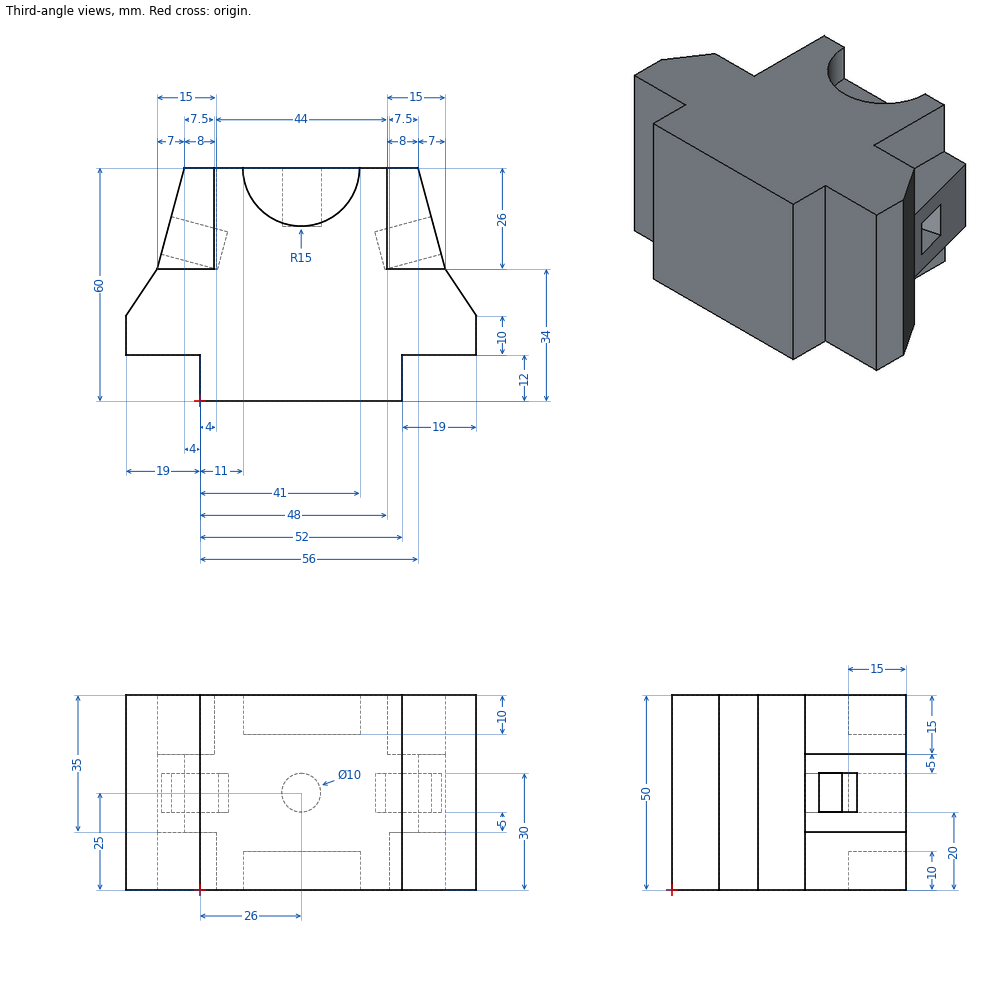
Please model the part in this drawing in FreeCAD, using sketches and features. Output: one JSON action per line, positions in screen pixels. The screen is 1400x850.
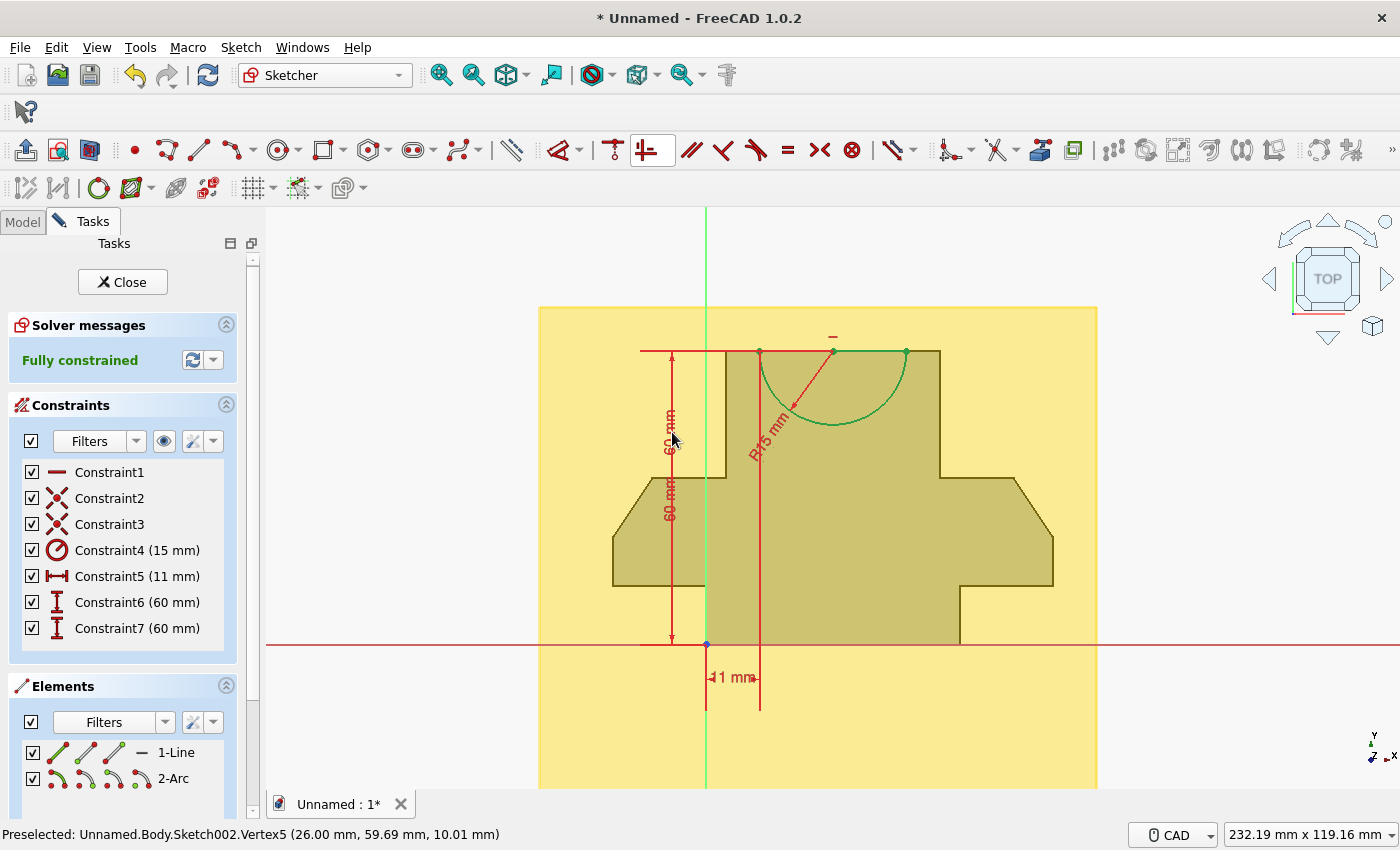
{"action": "left_click", "coordinate": [123, 282]}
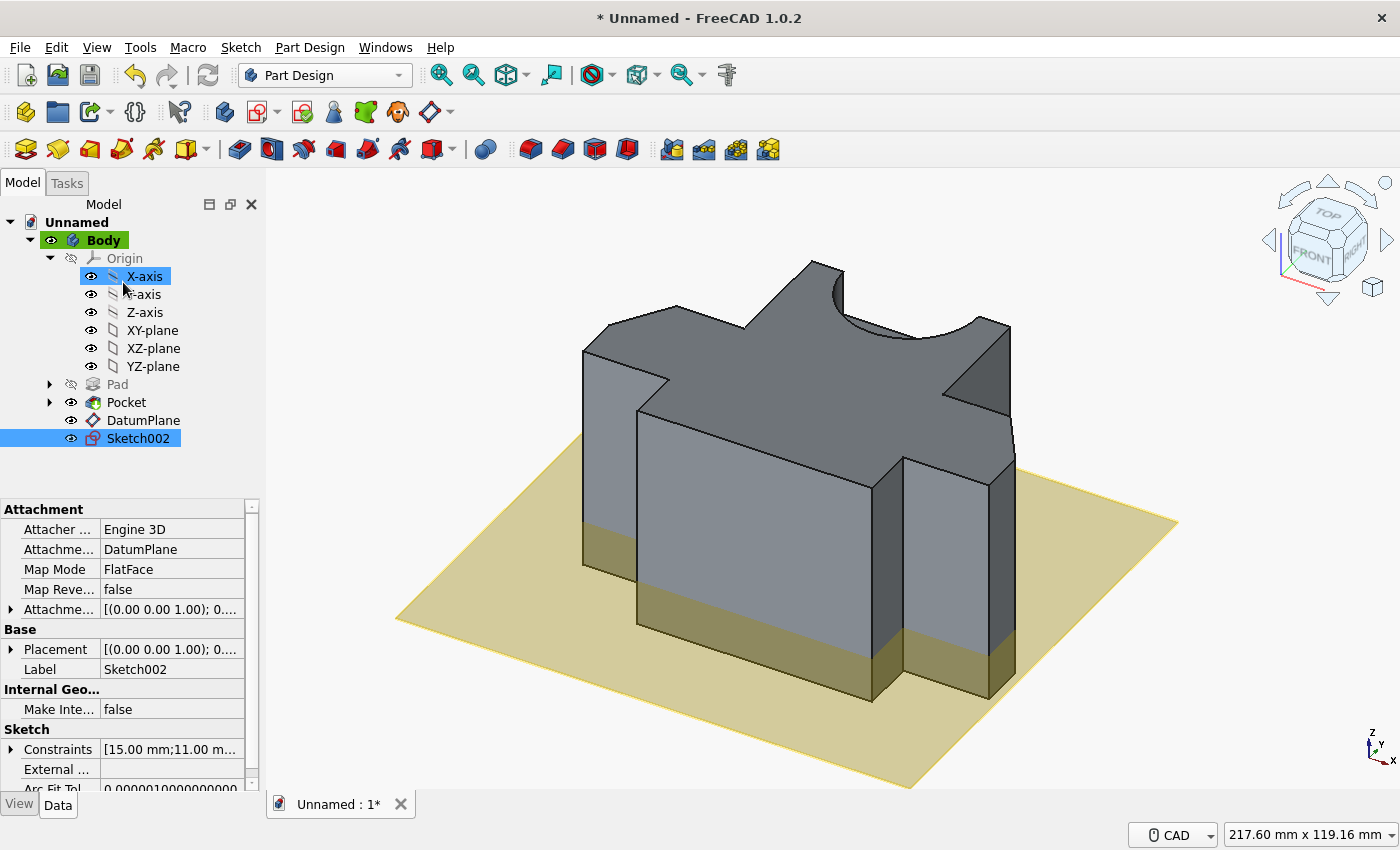
{"action": "left_click", "coordinate": [240, 150]}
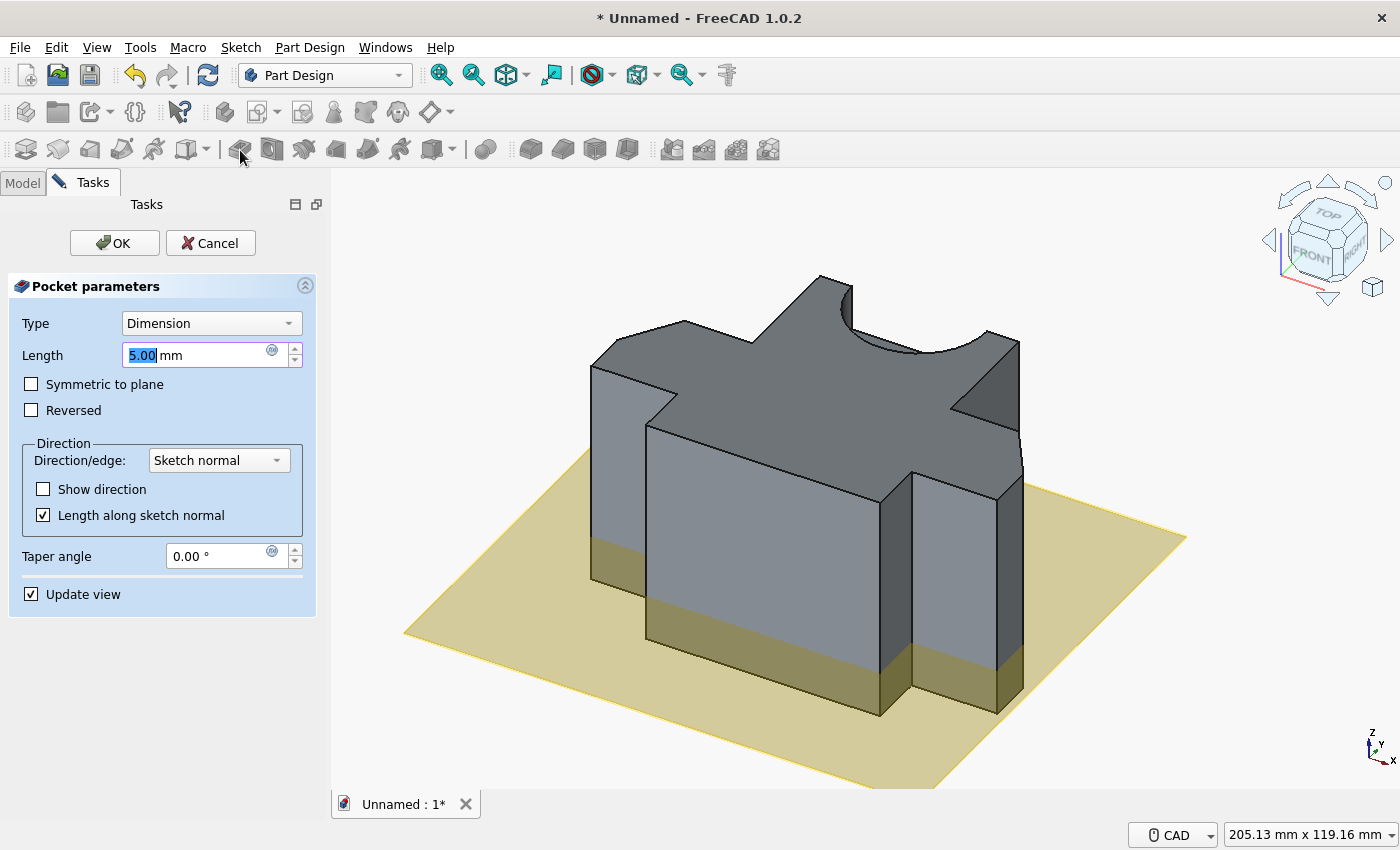
{"action": "type", "text": "10"}
{"action": "key", "text": "Tab"}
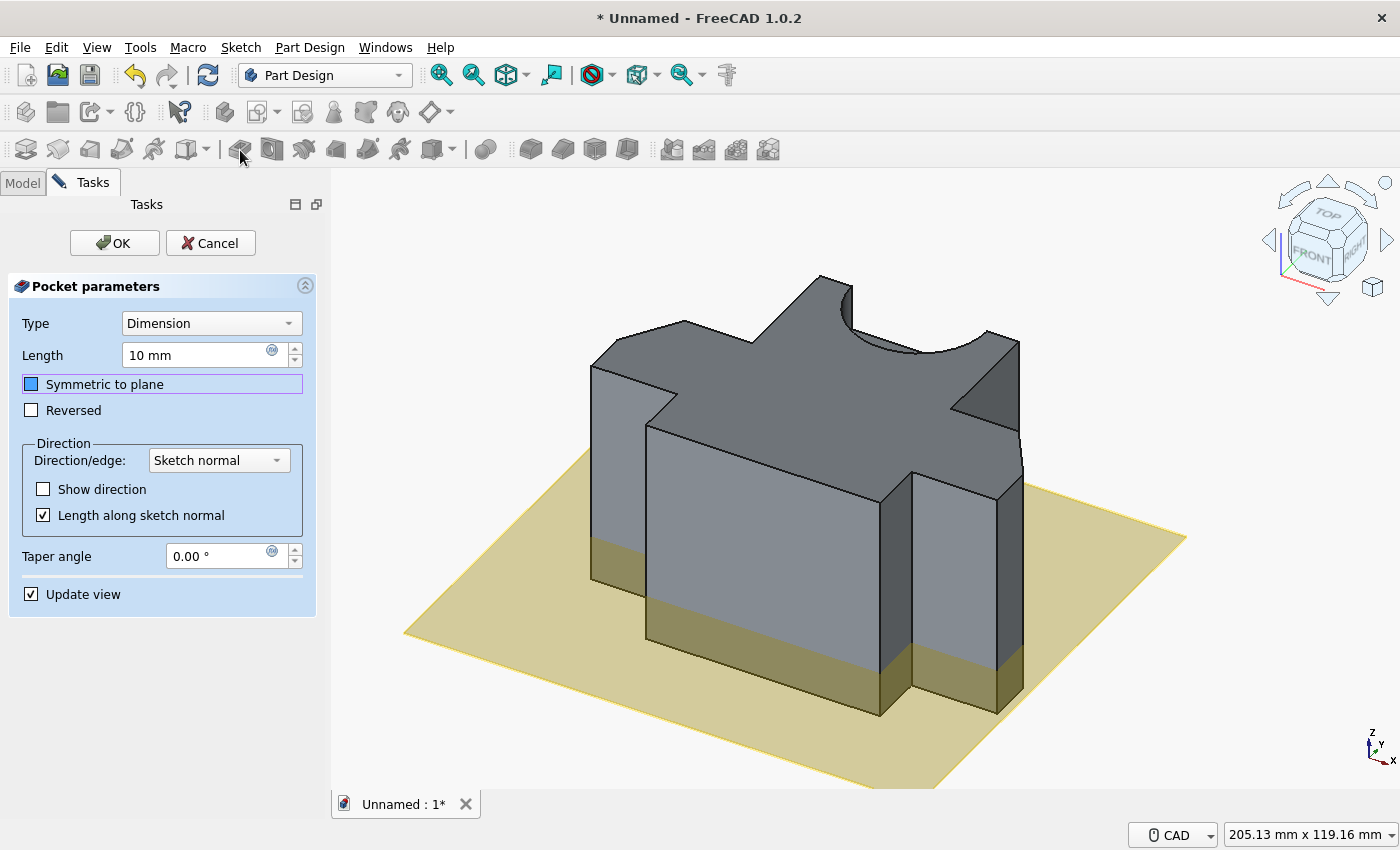
{"action": "left_click", "coordinate": [115, 243]}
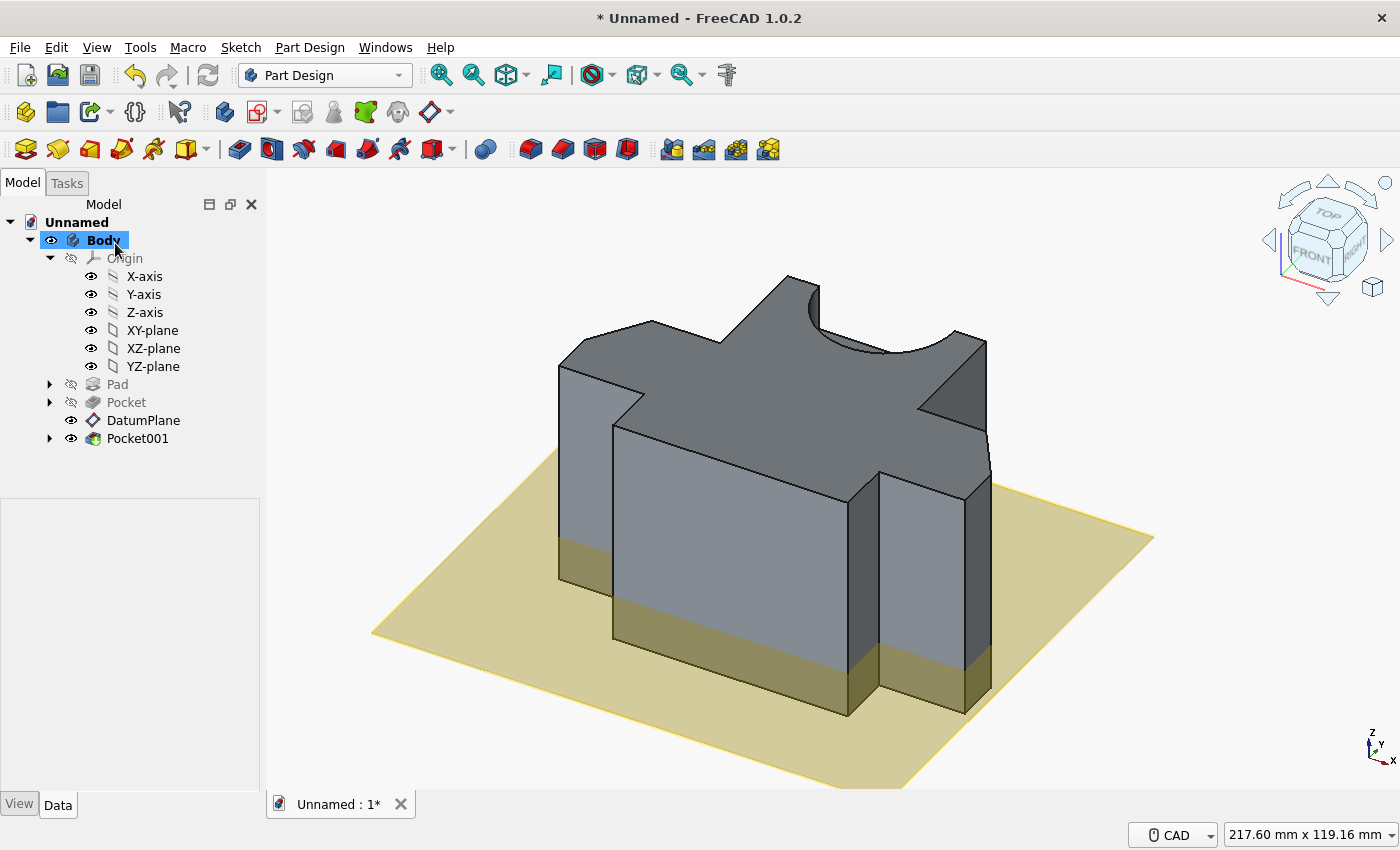
{"action": "left_click", "coordinate": [116, 420]}
{"action": "key", "text": "space"}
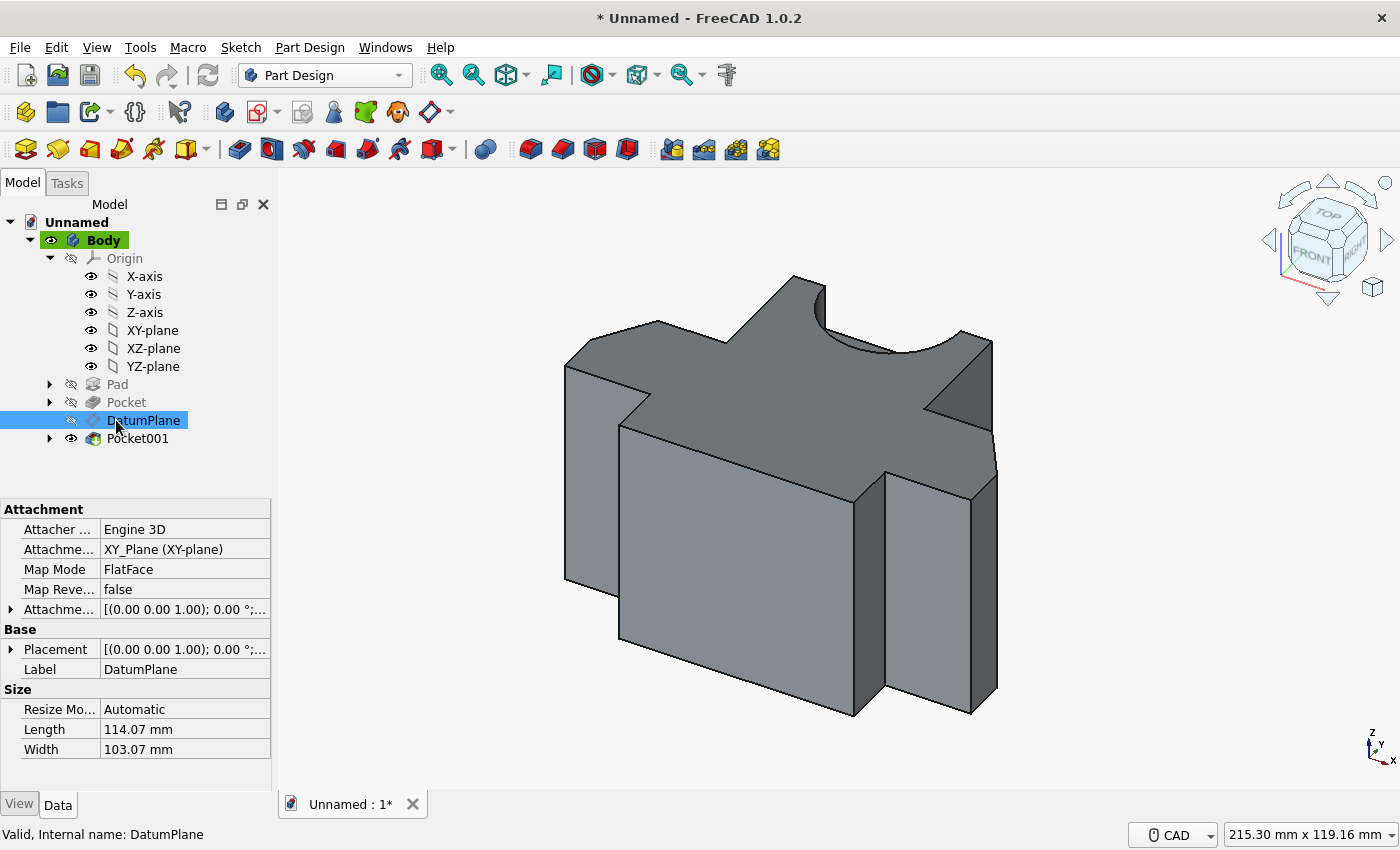
{"action": "left_click", "coordinate": [318, 749]}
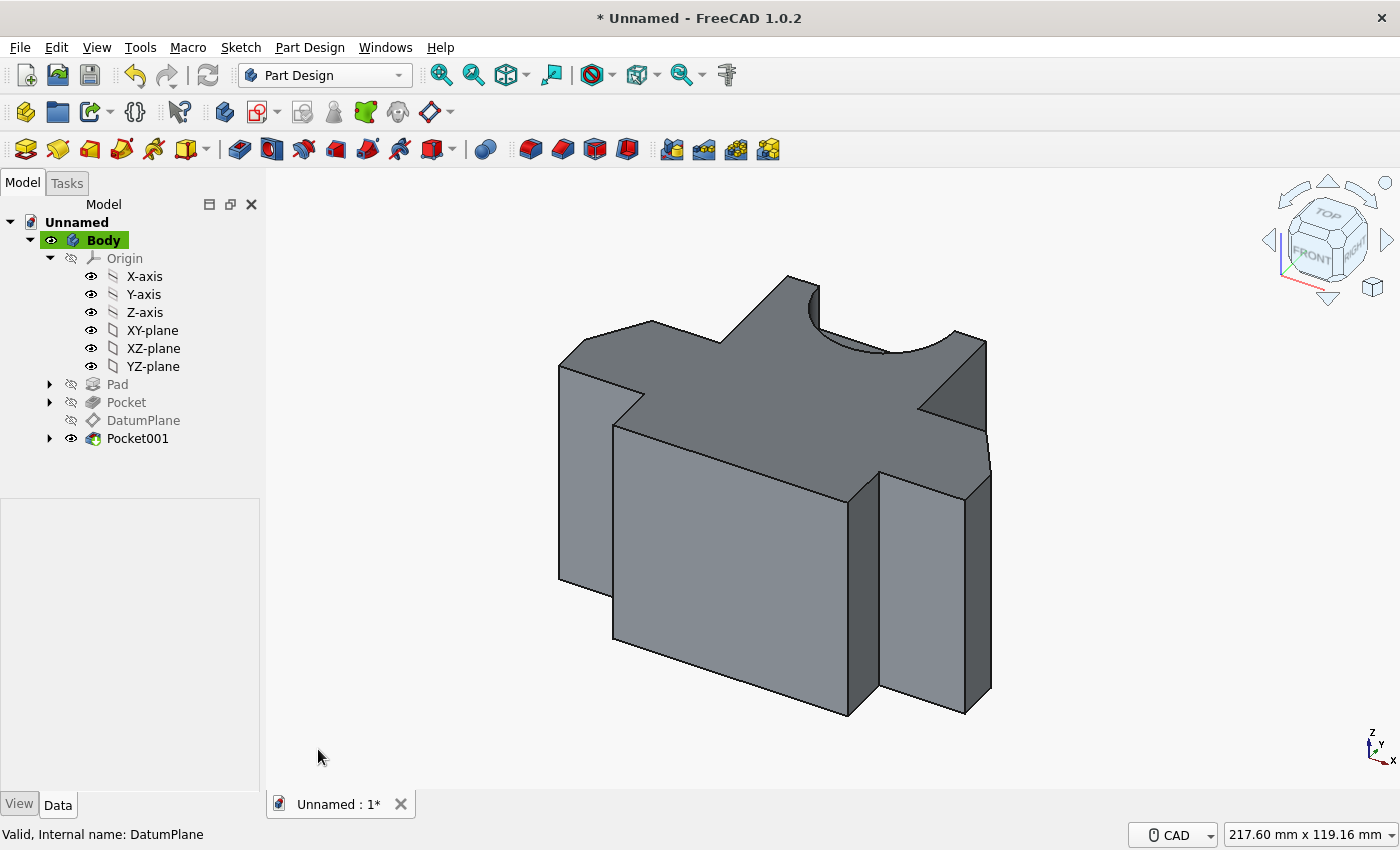
{"action": "left_click", "coordinate": [258, 112]}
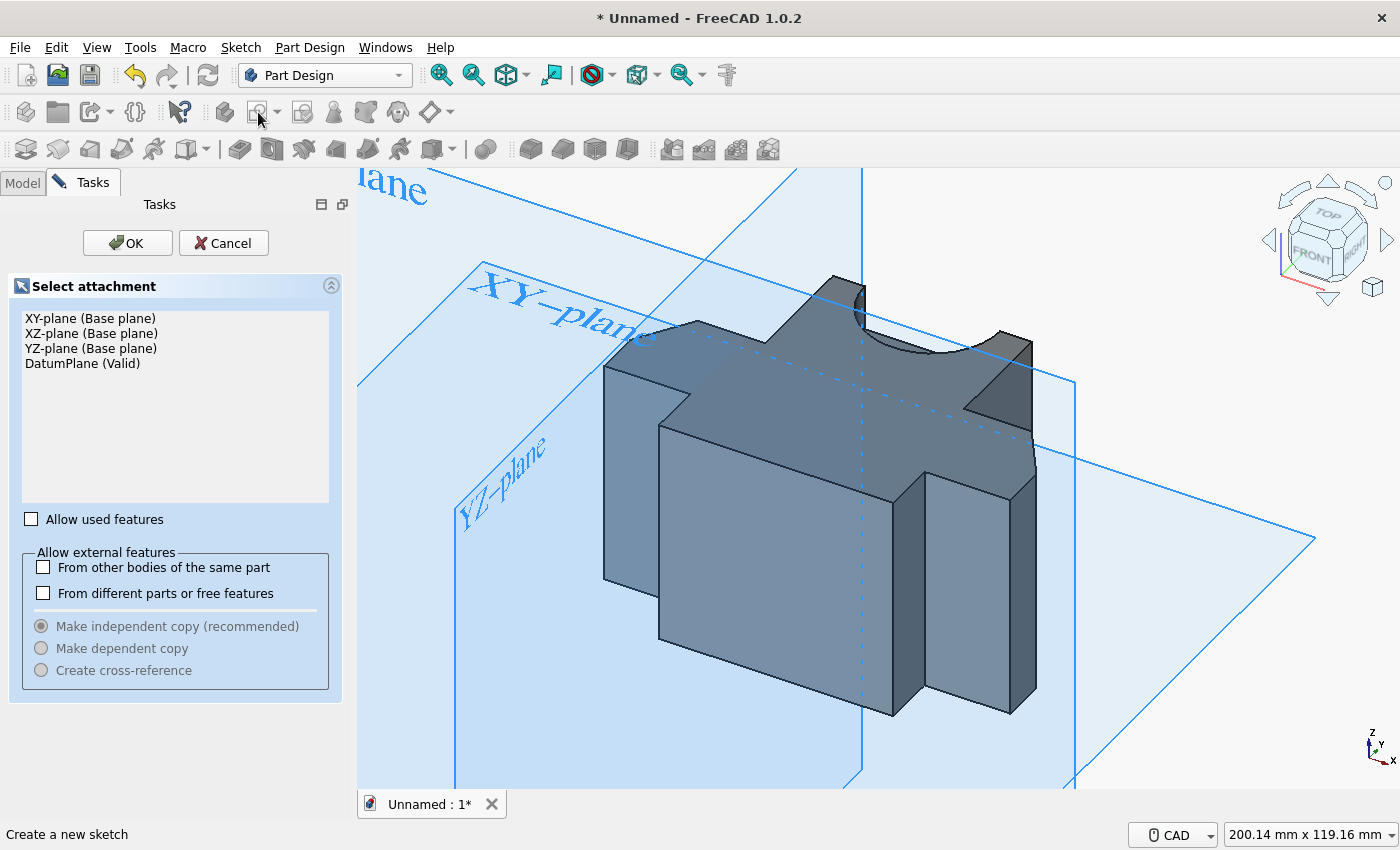
{"action": "left_click", "coordinate": [82, 318]}